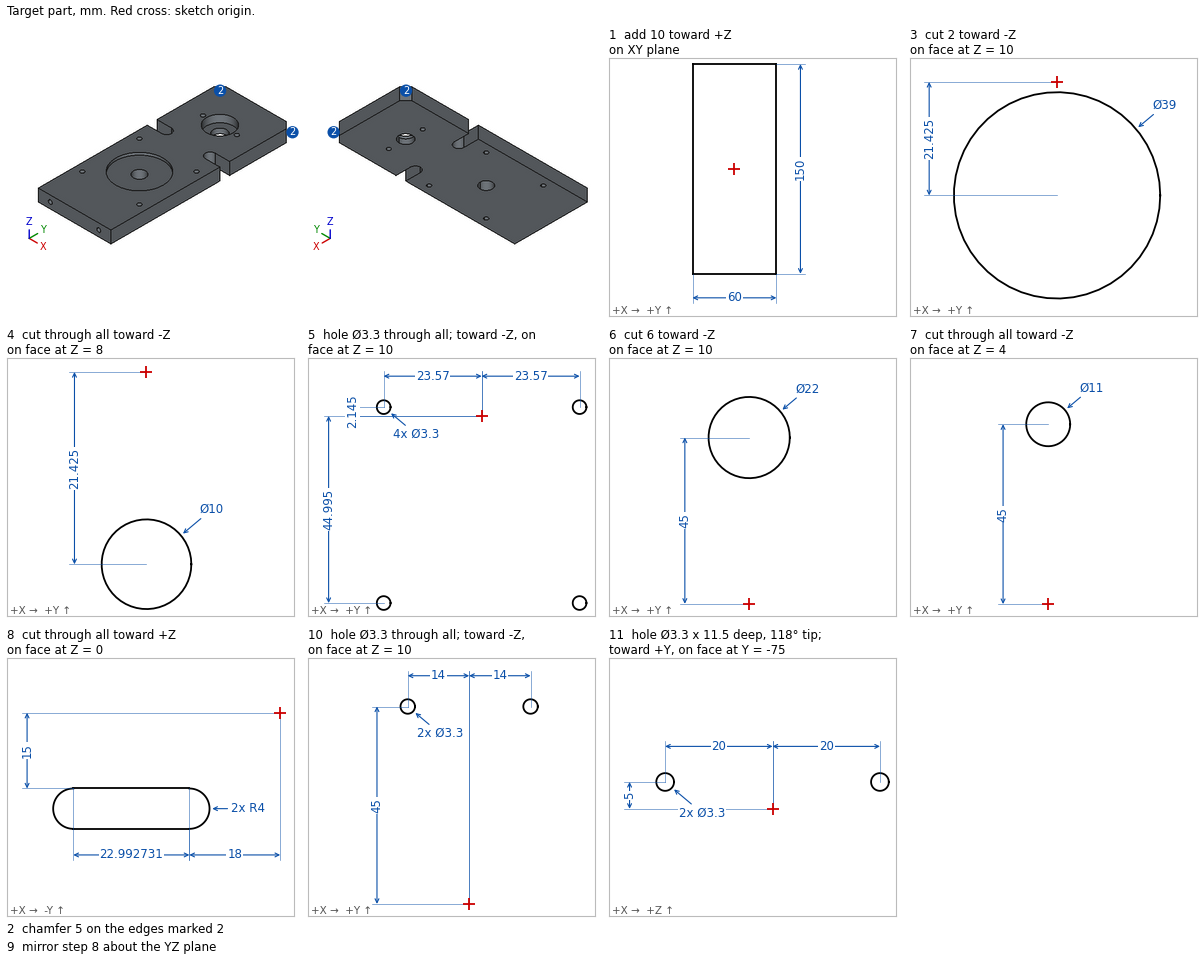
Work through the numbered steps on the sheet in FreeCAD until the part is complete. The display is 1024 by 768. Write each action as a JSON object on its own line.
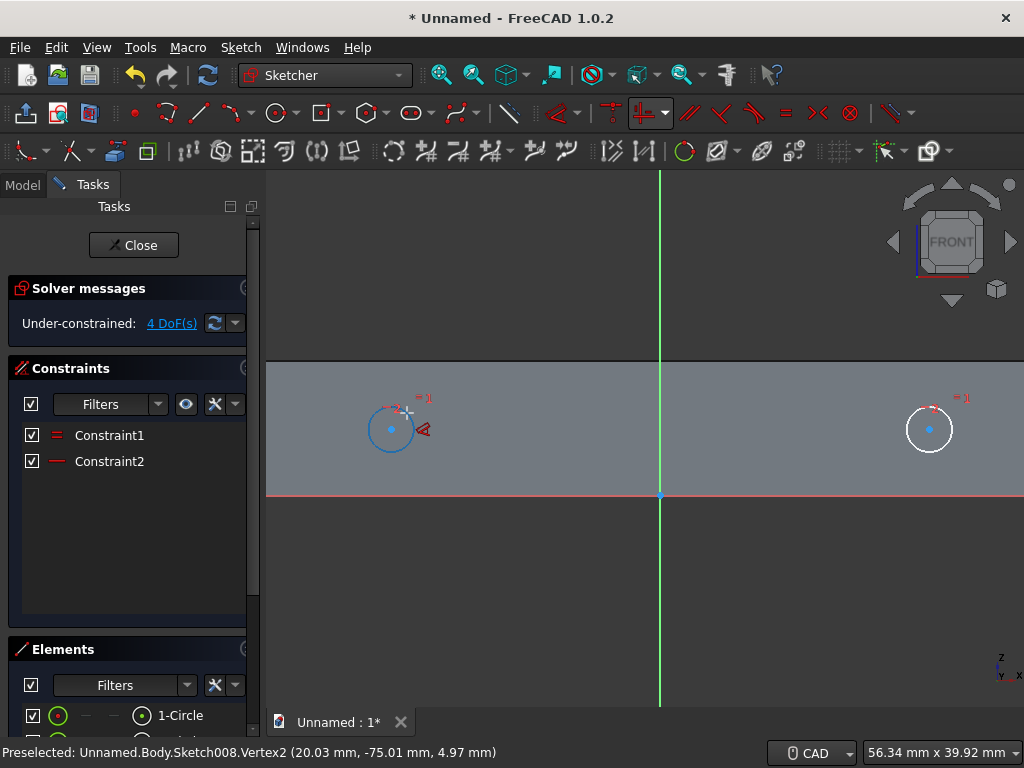
{"action": "left_click", "coordinate": [407, 413]}
{"action": "left_click", "coordinate": [429, 390]}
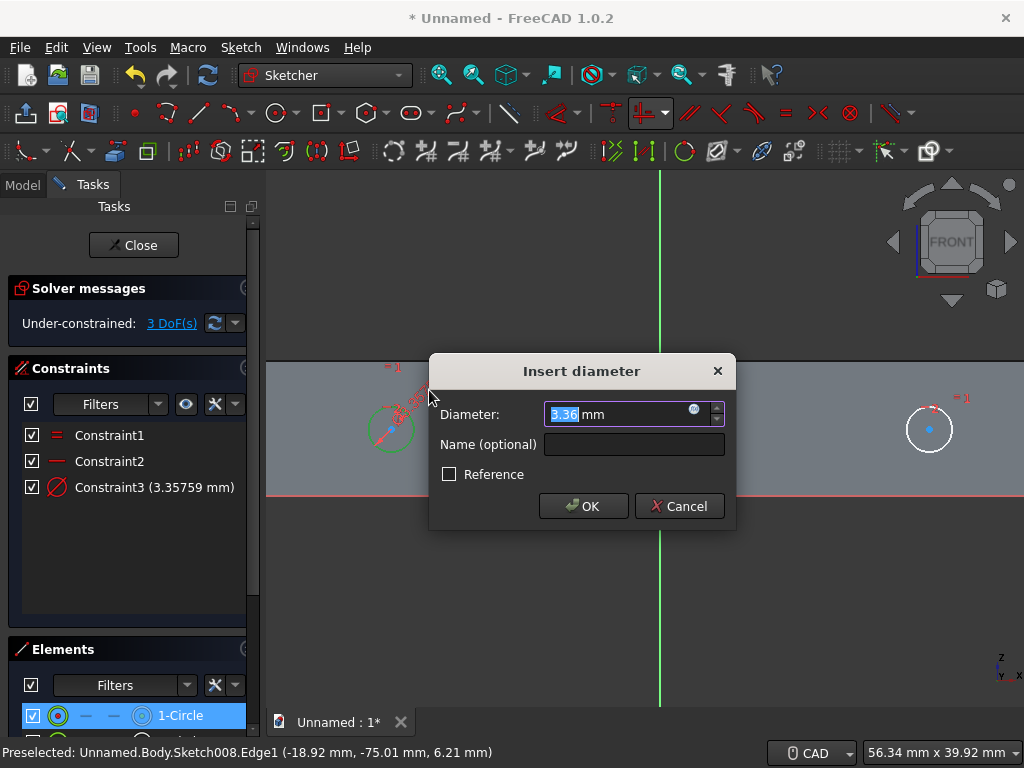
{"action": "type", "text": "3.3"}
{"action": "key", "text": "Return"}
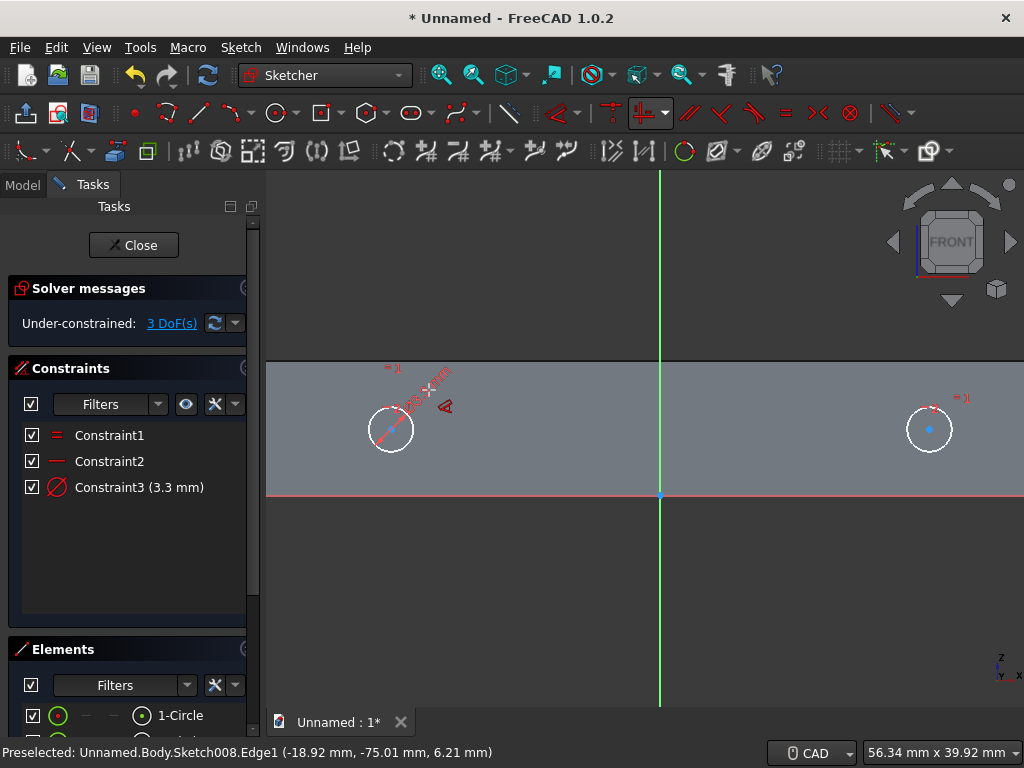
{"action": "left_click", "coordinate": [391, 430]}
{"action": "left_click", "coordinate": [357, 463]}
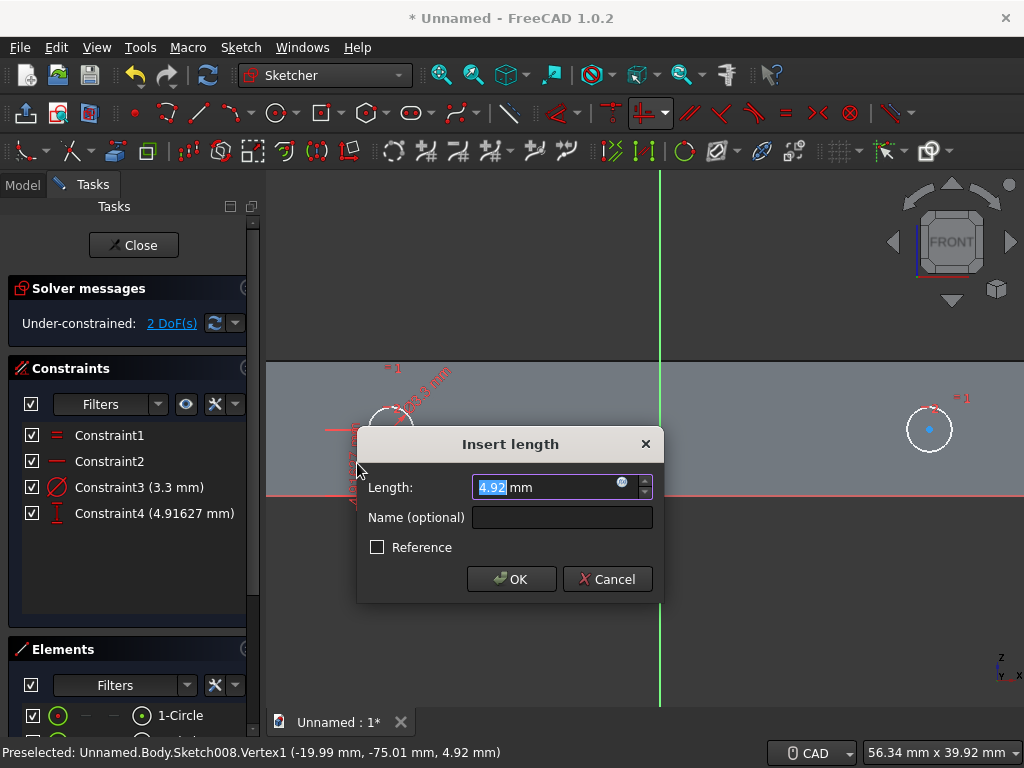
{"action": "type", "text": "5"}
{"action": "key", "text": "Return"}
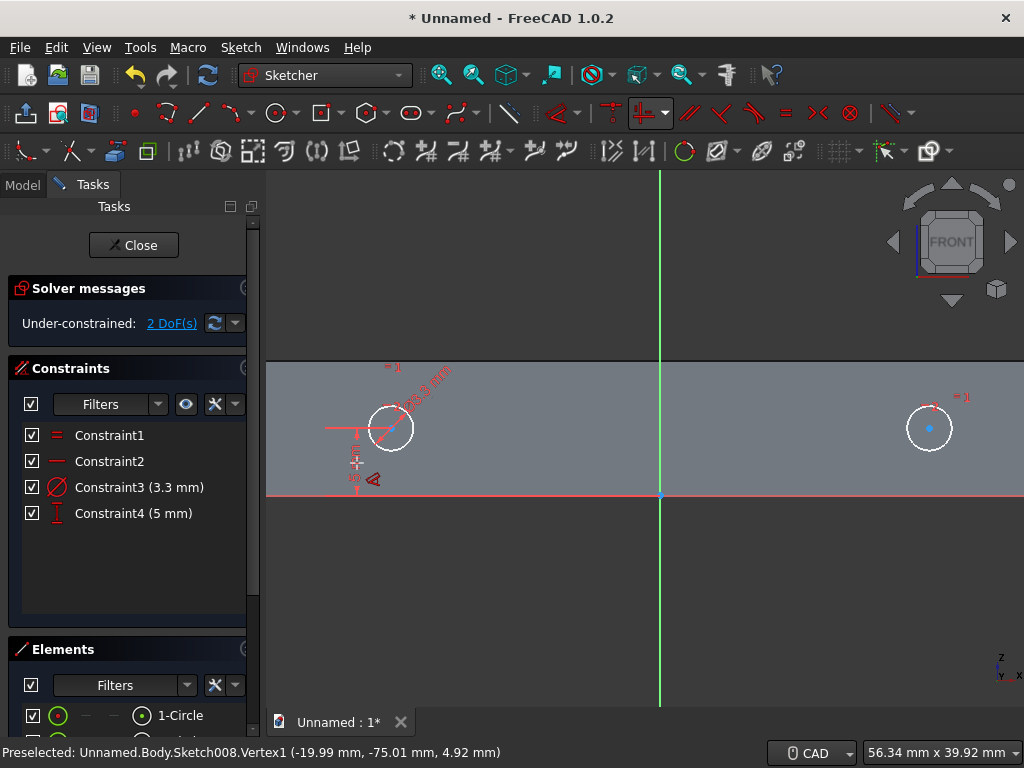
{"action": "left_click", "coordinate": [391, 428]}
{"action": "left_click", "coordinate": [526, 530]}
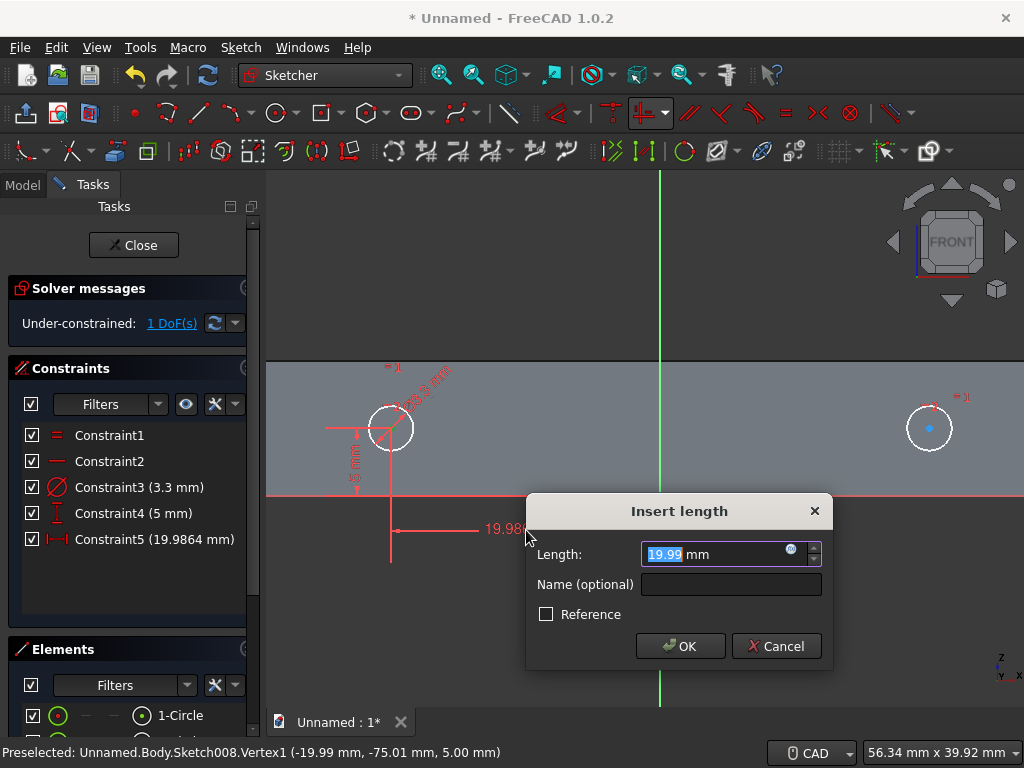
{"action": "type", "text": "20"}
{"action": "key", "text": "Return"}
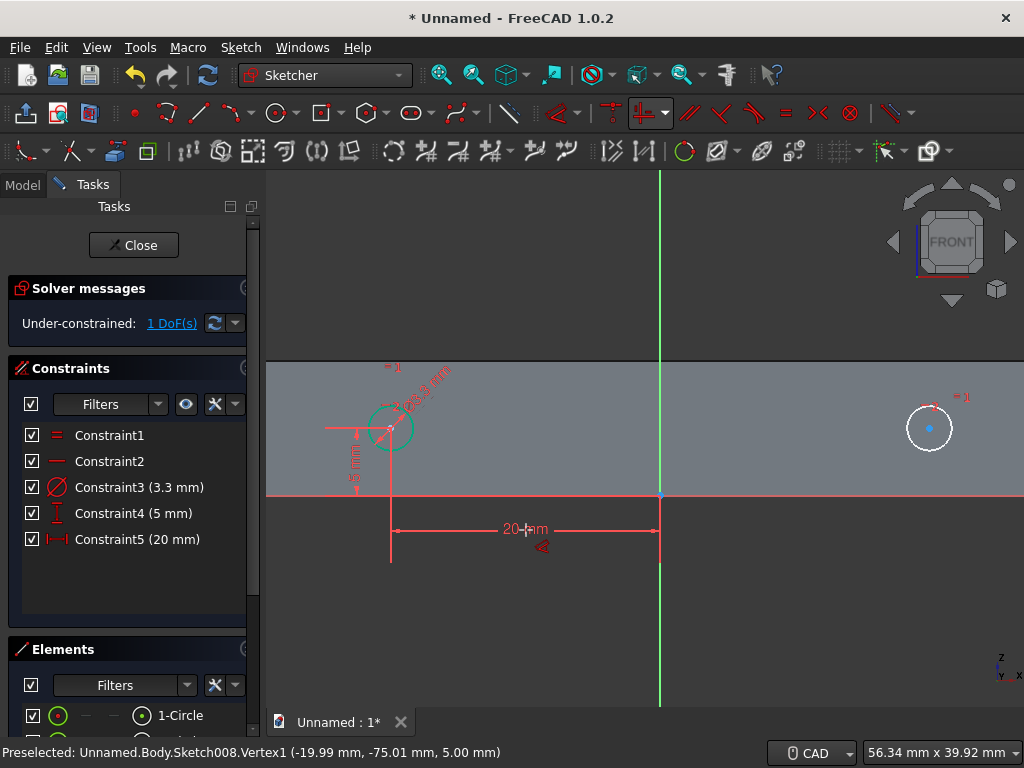
{"action": "scroll", "coordinate": [407, 413], "scroll_direction": "down", "scroll_amount": 2}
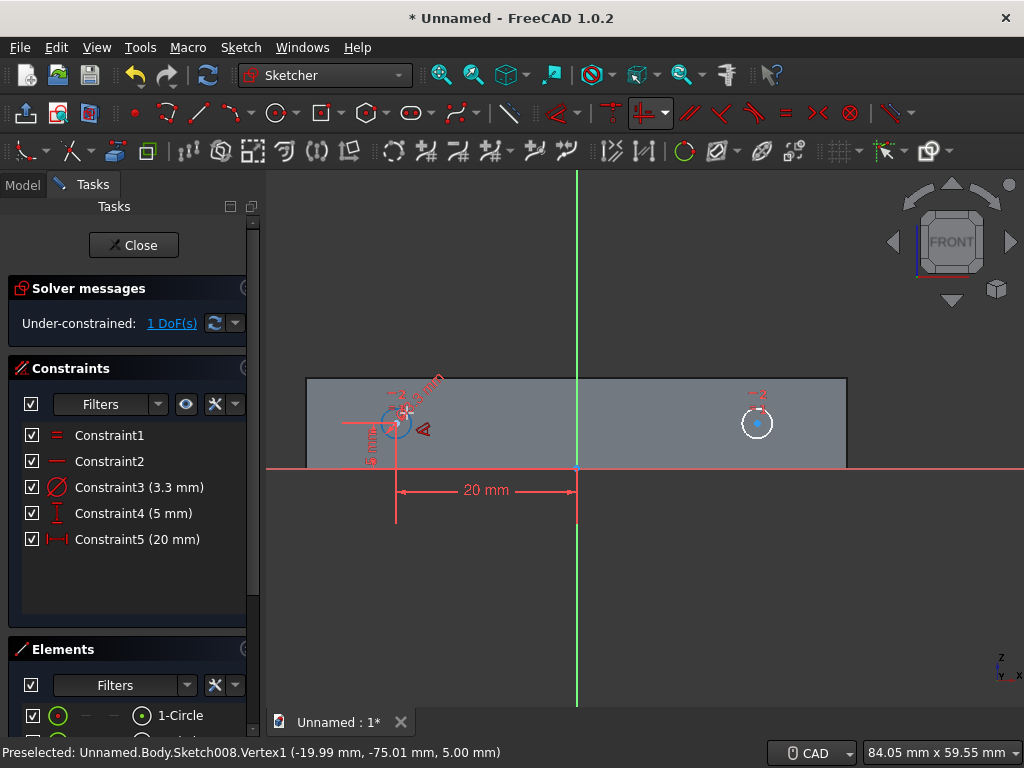
{"action": "left_click", "coordinate": [757, 423]}
{"action": "left_click", "coordinate": [667, 503]}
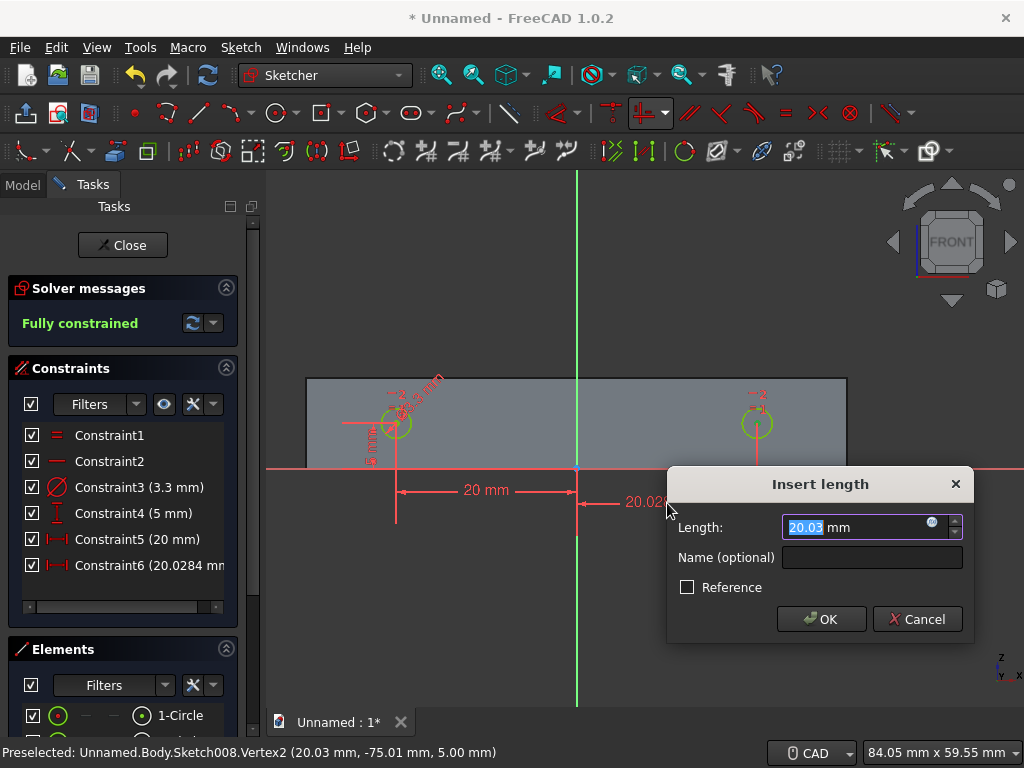
{"action": "type", "text": "20"}
{"action": "key", "text": "Return"}
{"action": "key", "text": "Escape"}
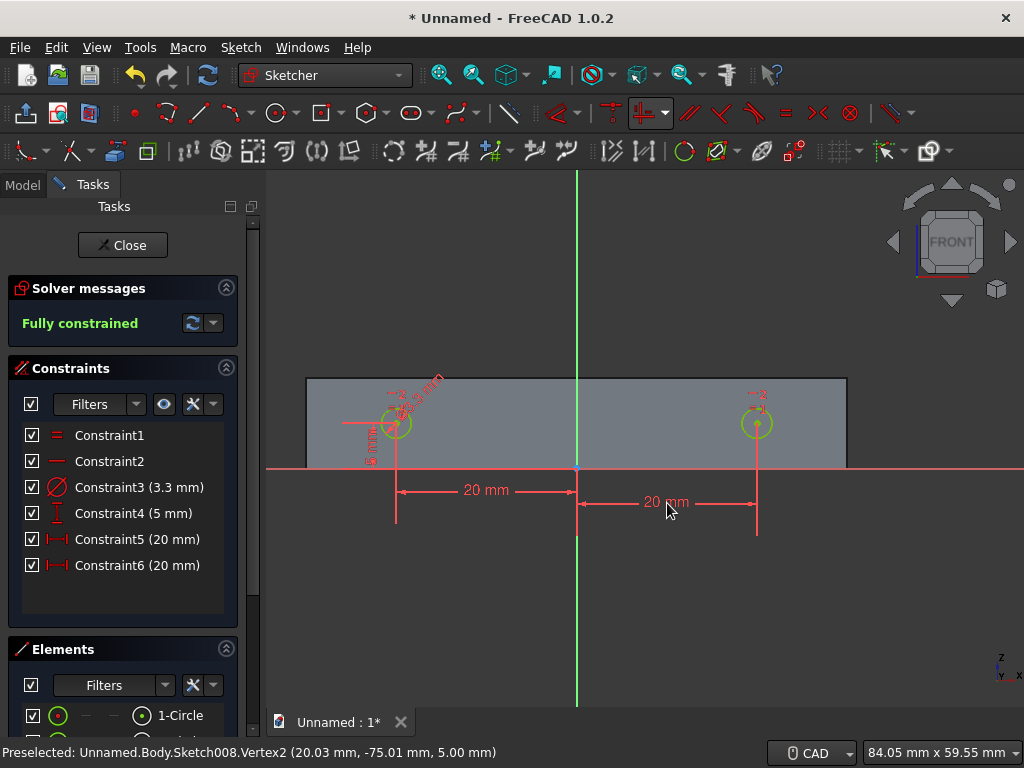
{"action": "left_click", "coordinate": [123, 245]}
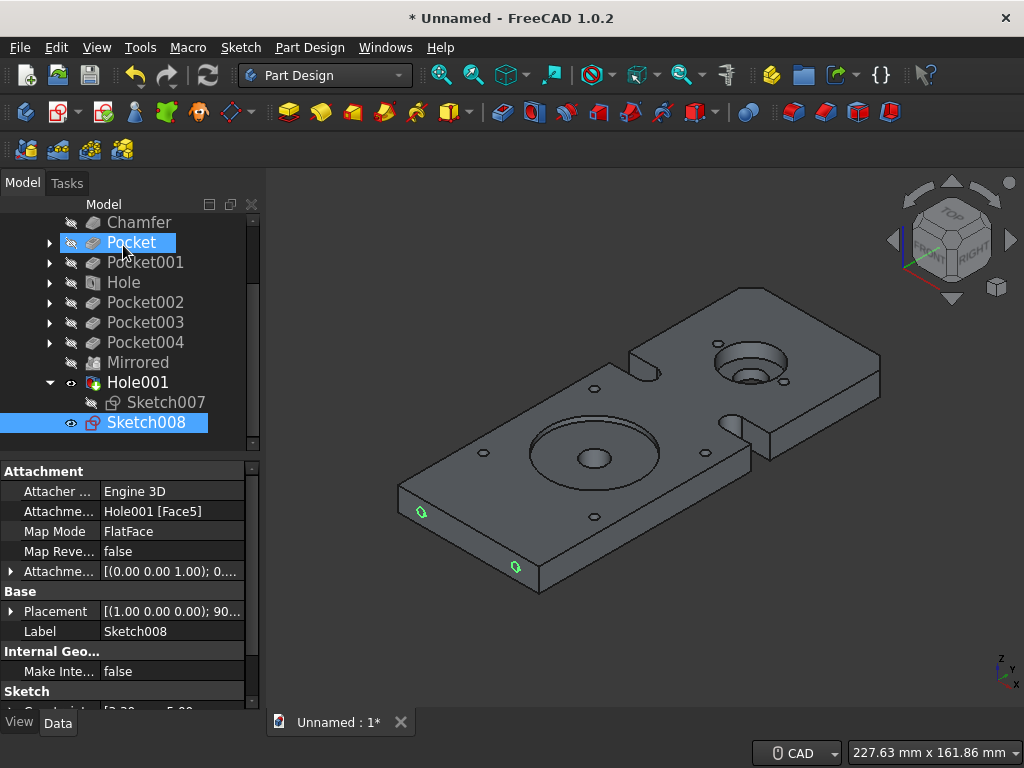
{"action": "left_click", "coordinate": [536, 112]}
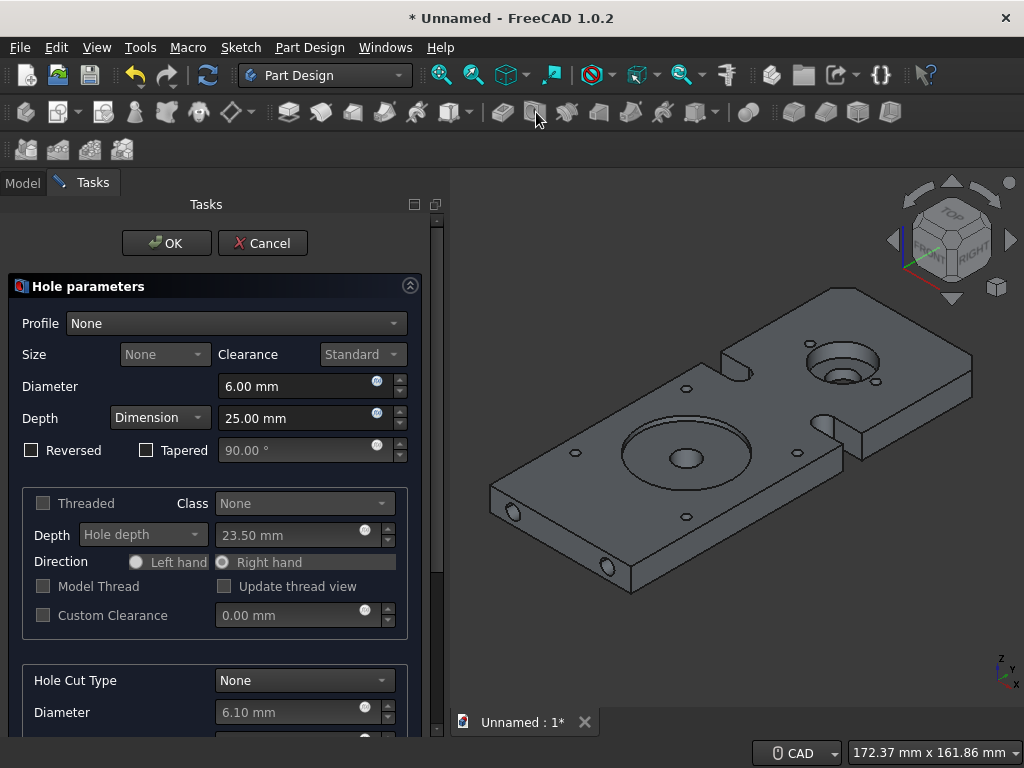
{"action": "triple_click", "coordinate": [305, 386]}